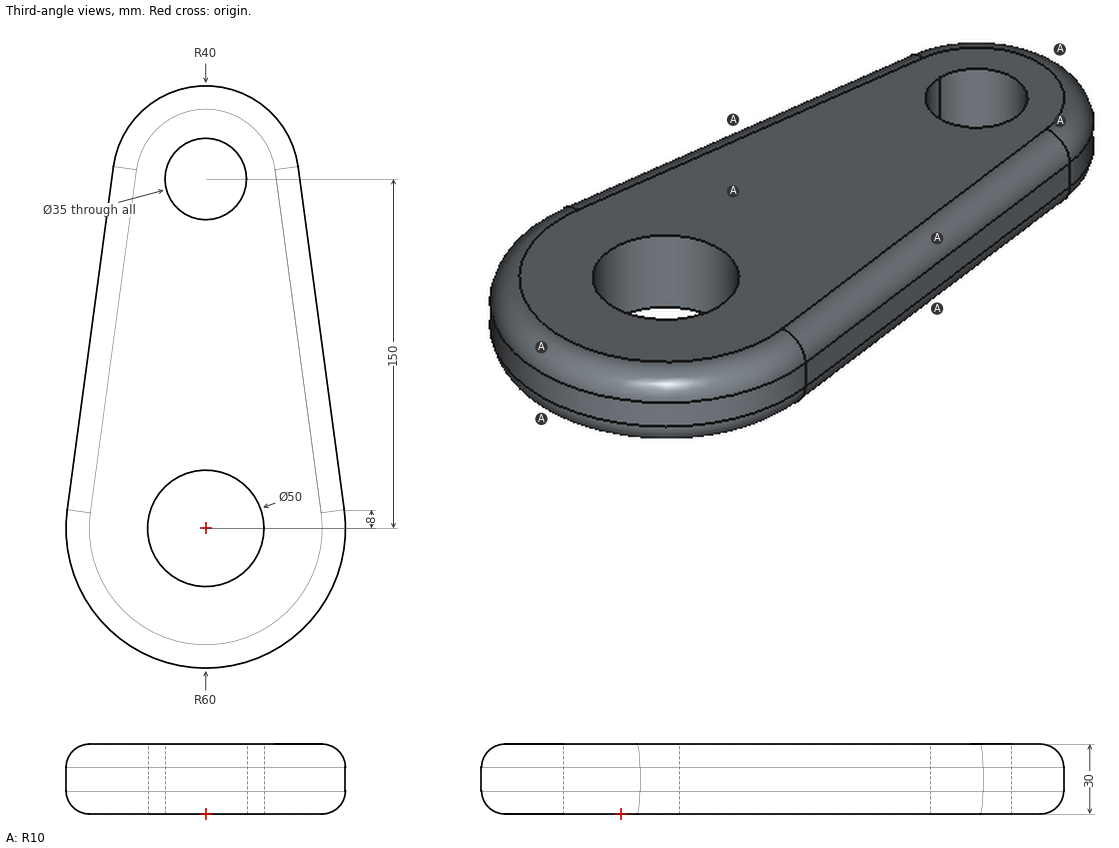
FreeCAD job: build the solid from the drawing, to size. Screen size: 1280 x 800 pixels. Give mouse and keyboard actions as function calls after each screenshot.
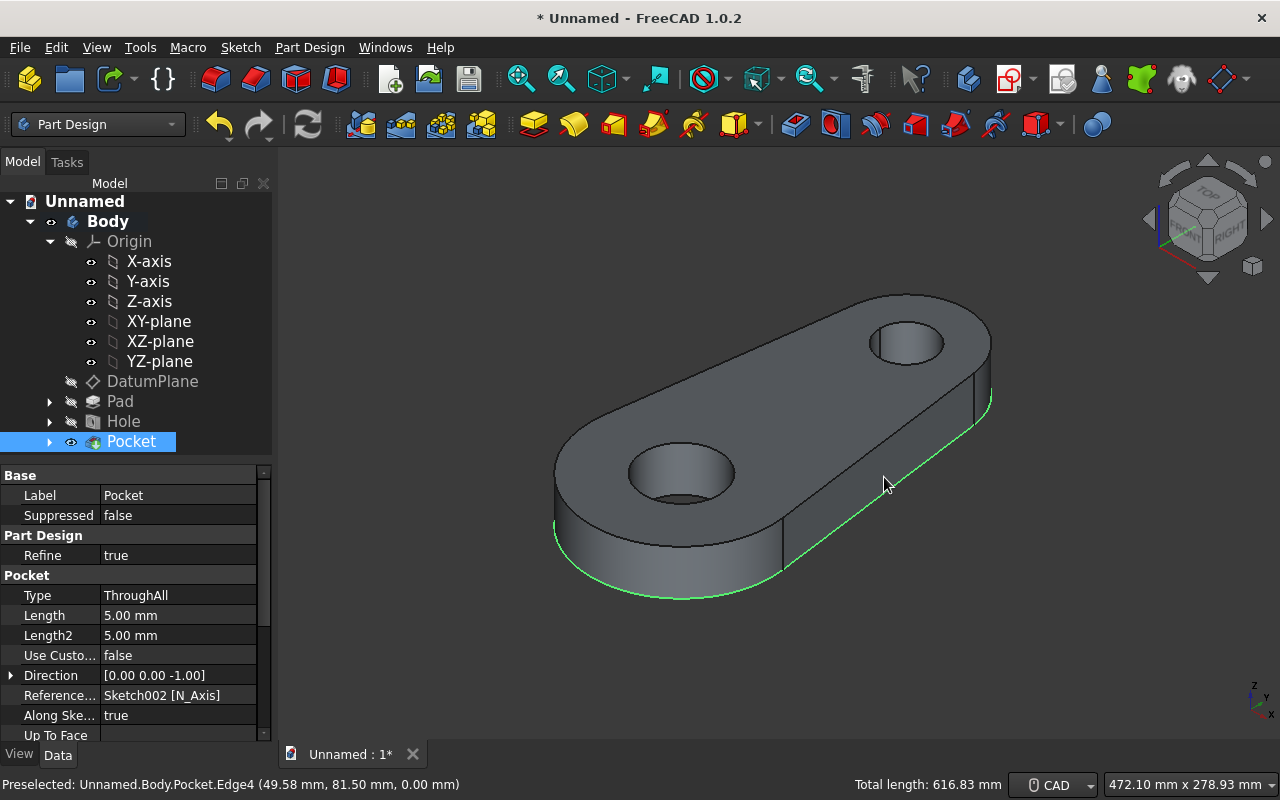
click(981, 319, ctrl)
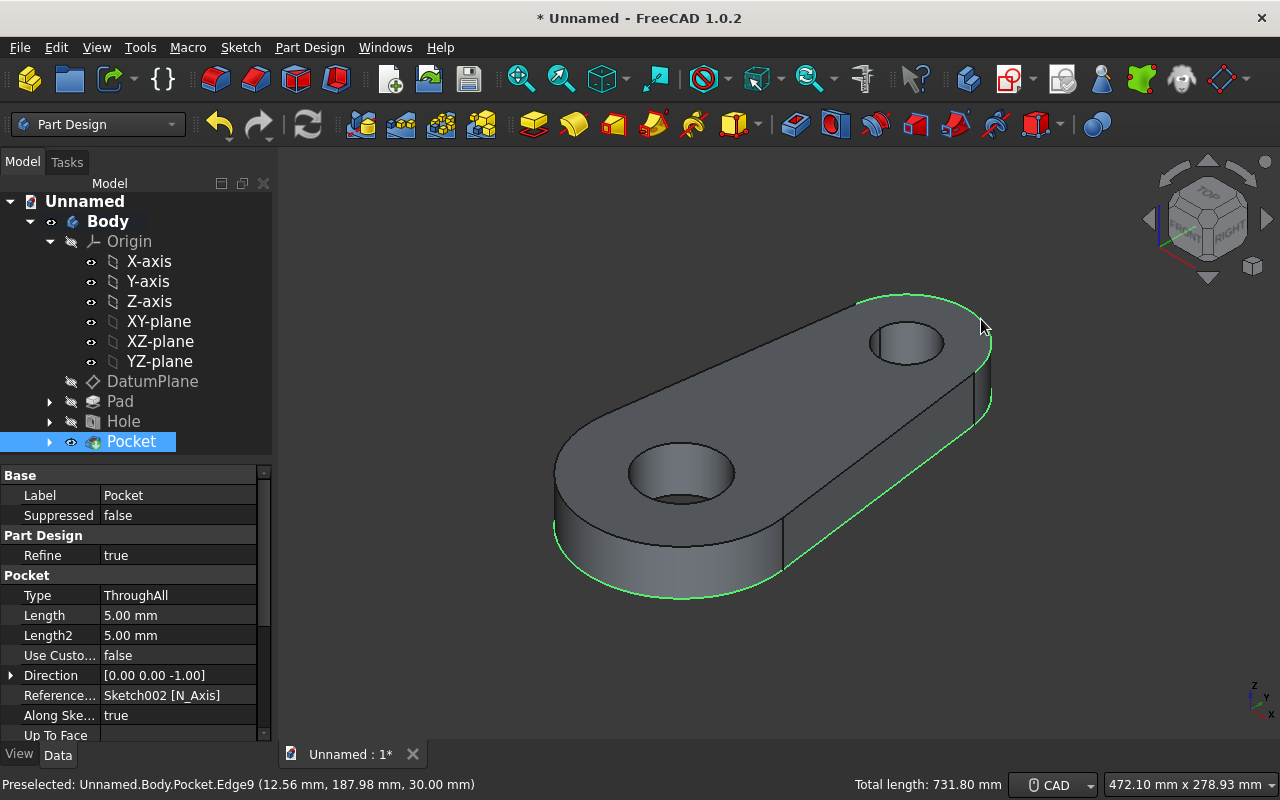
click(878, 445, ctrl)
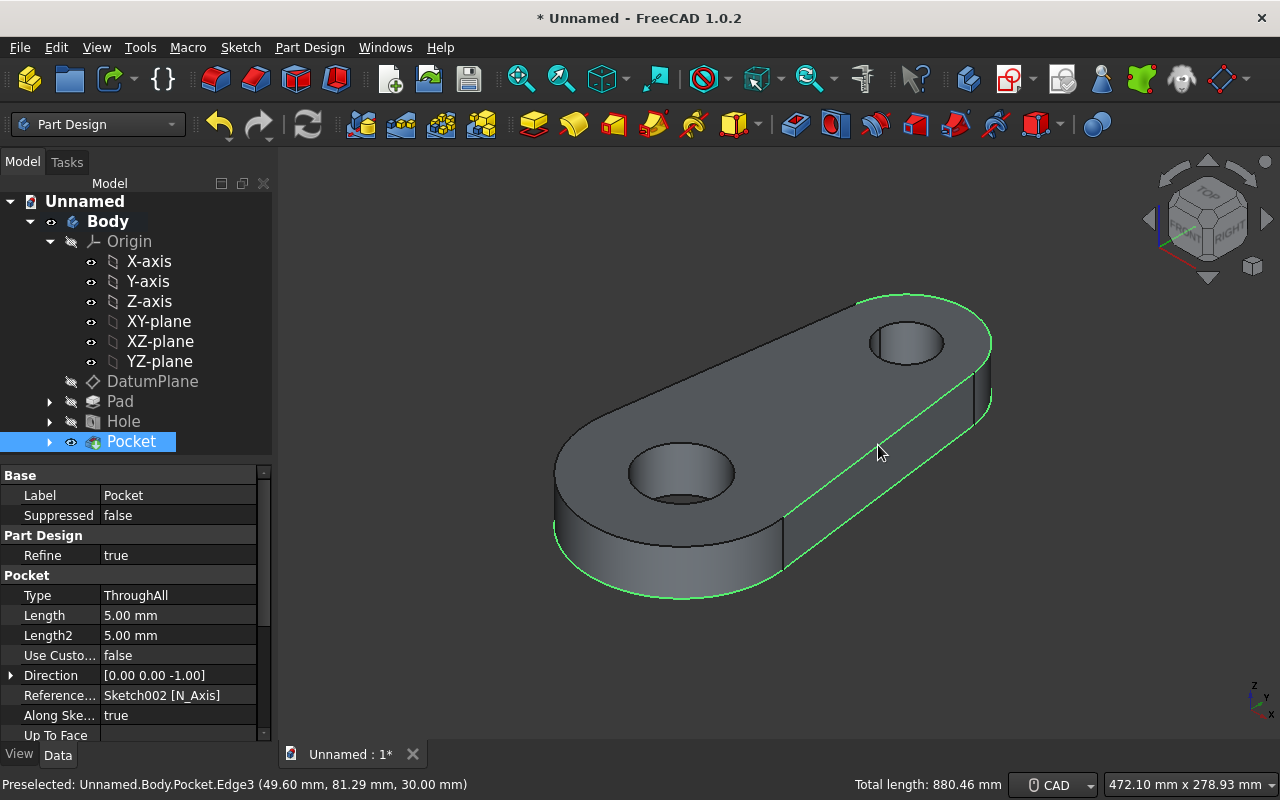
click(591, 524, ctrl)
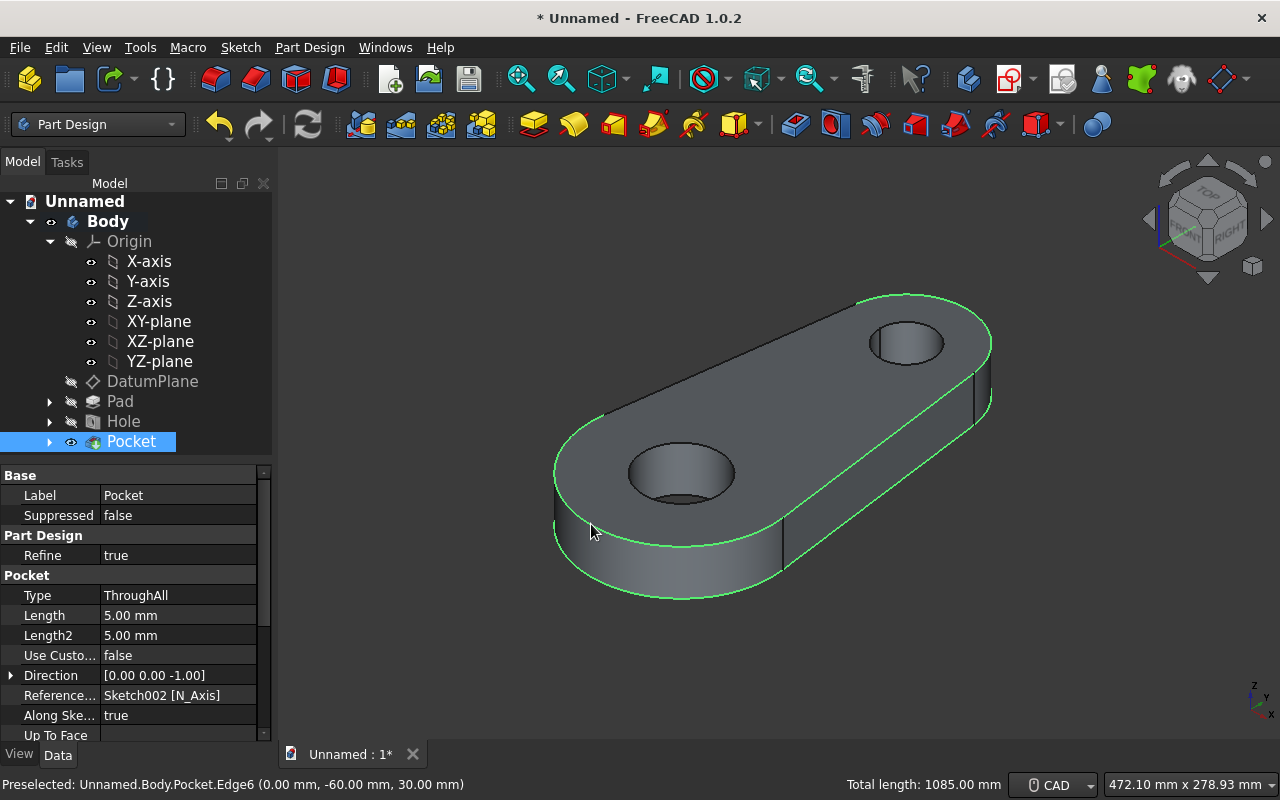
key(2)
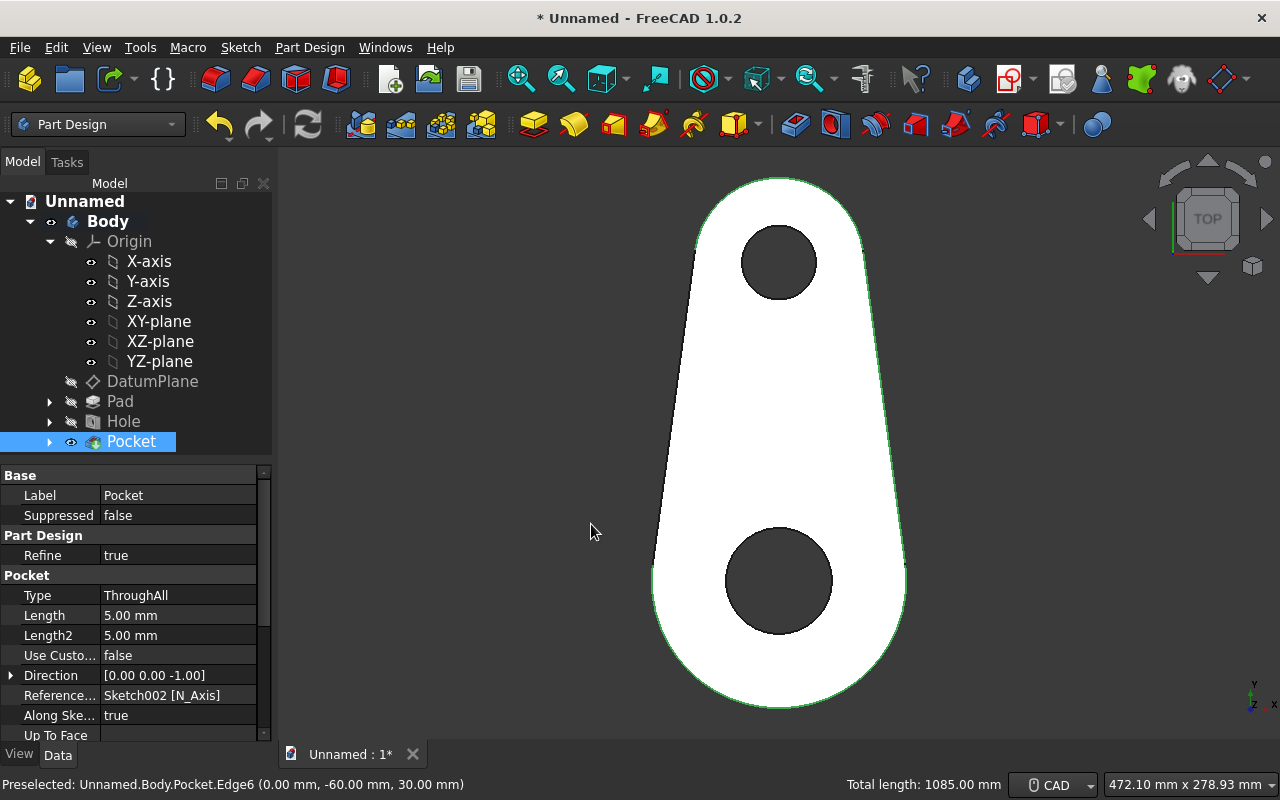
click(674, 407, ctrl)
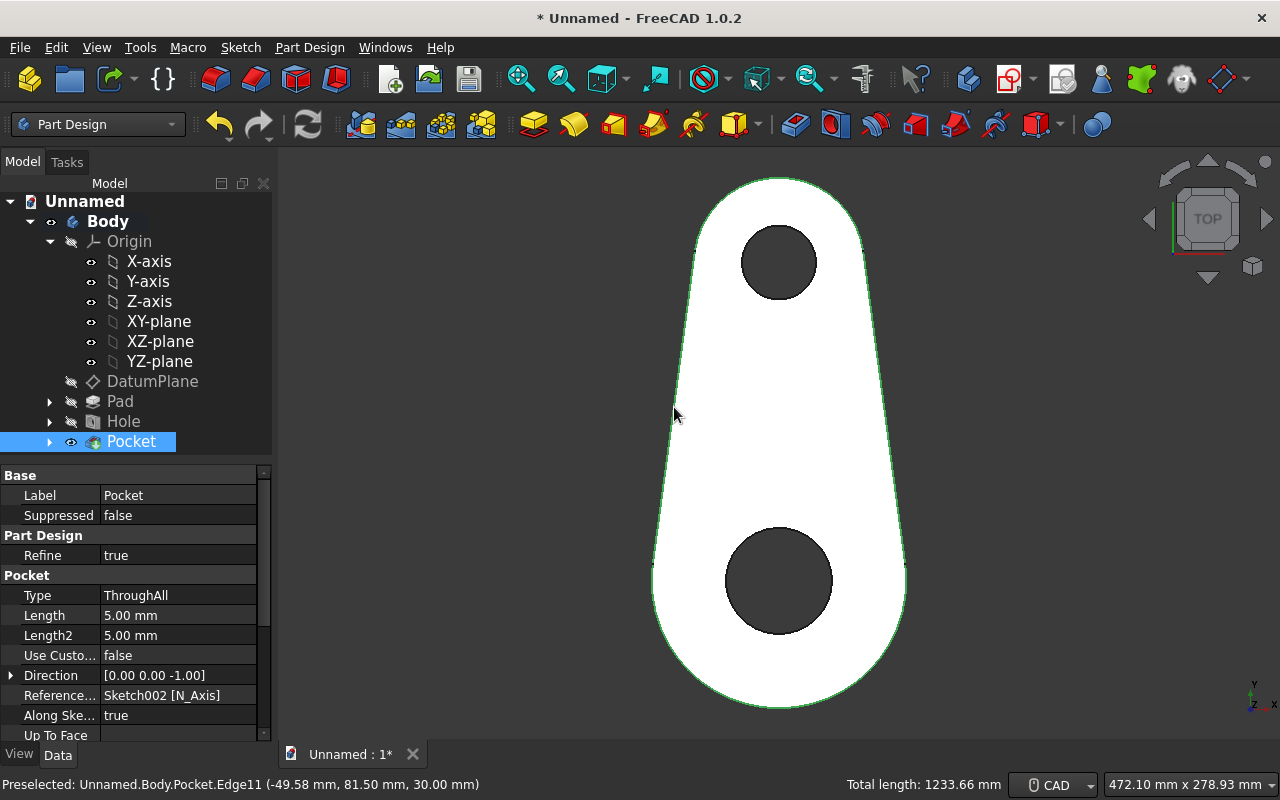
click(216, 80)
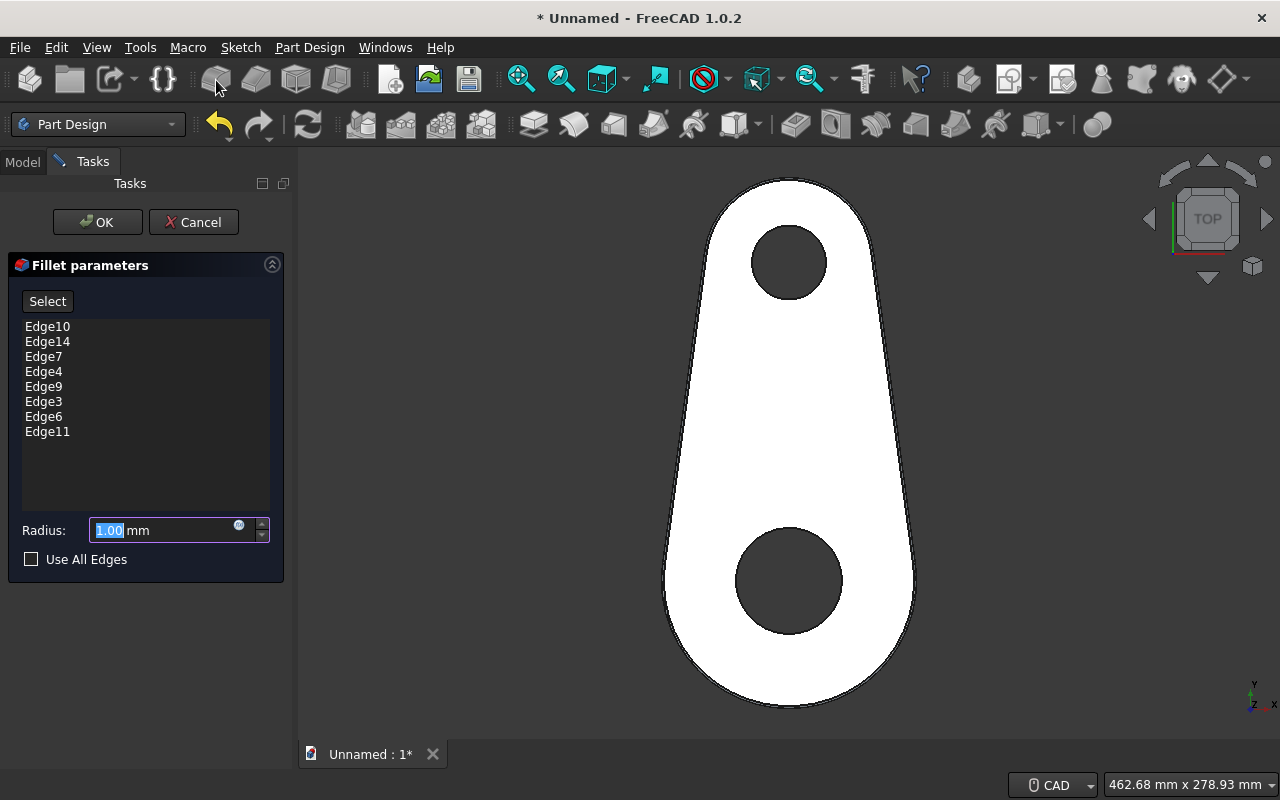
text(10)
key(Tab)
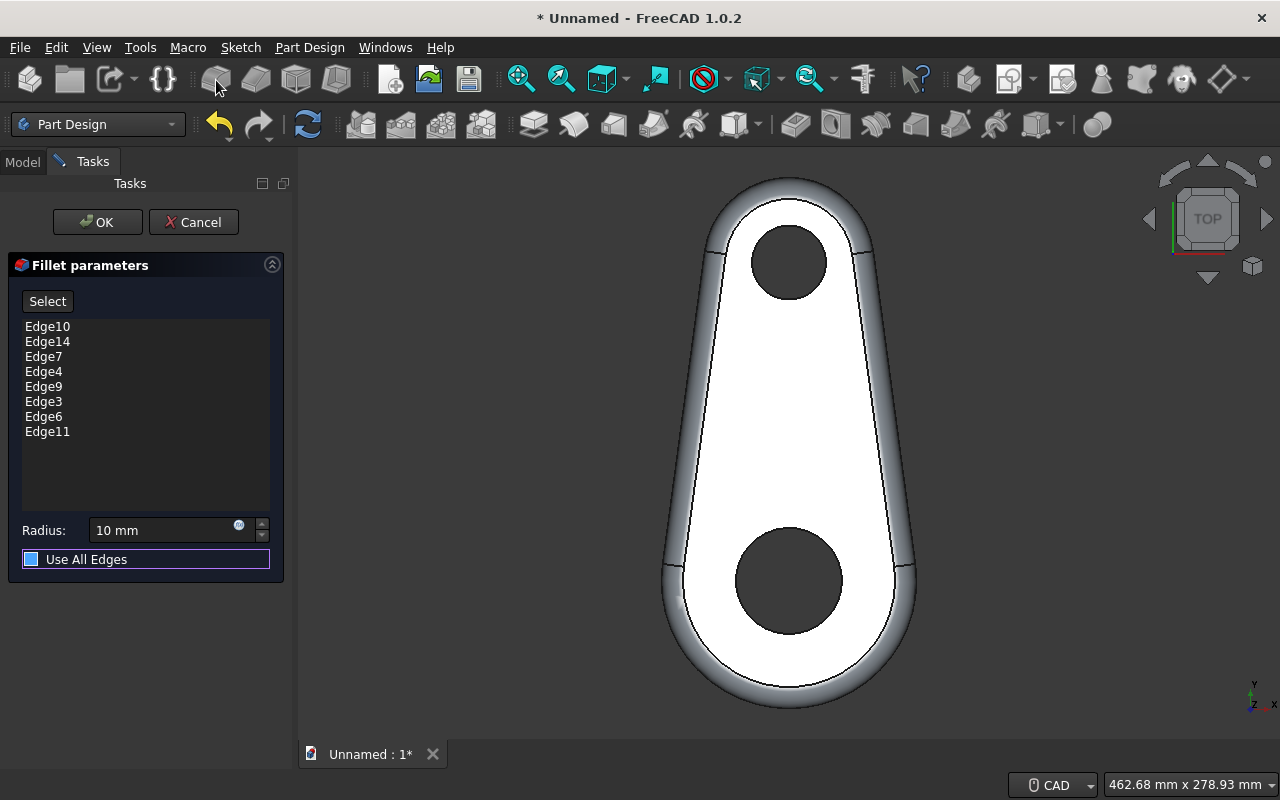
click(98, 222)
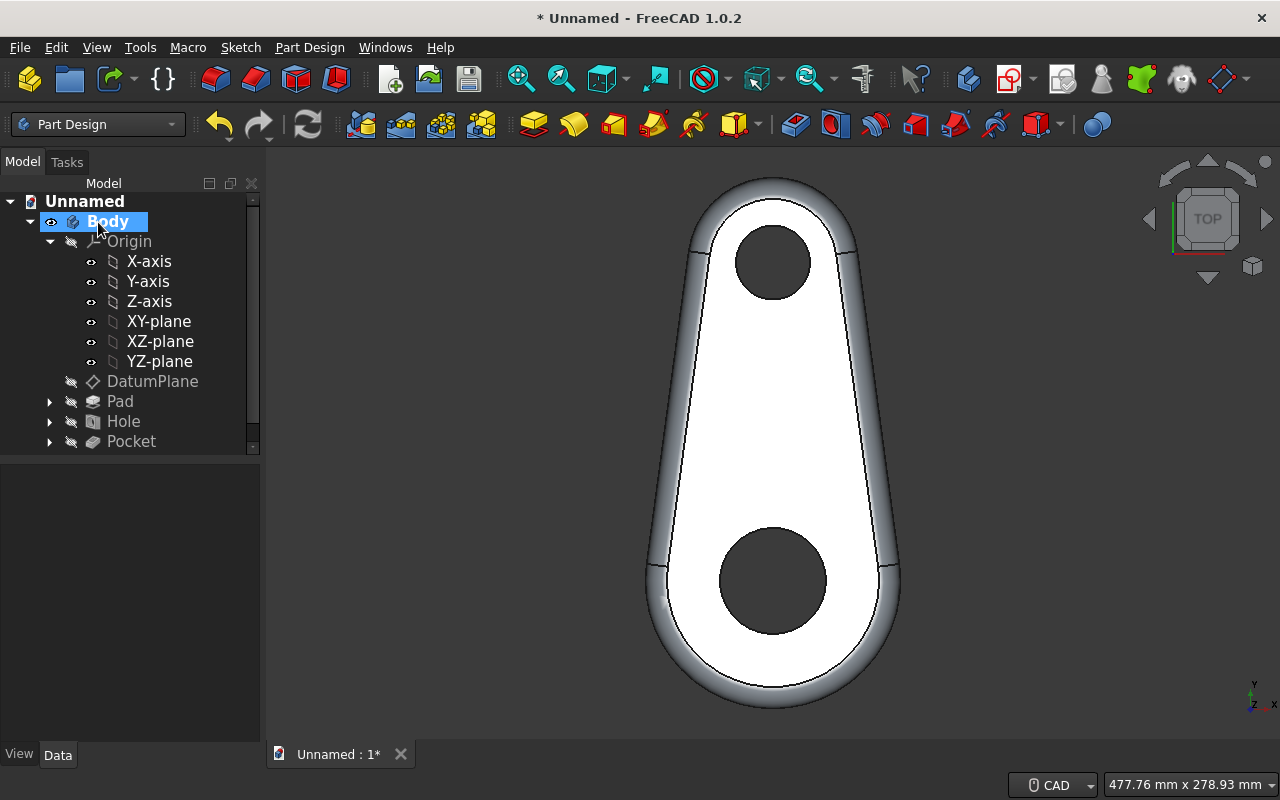
key(0)